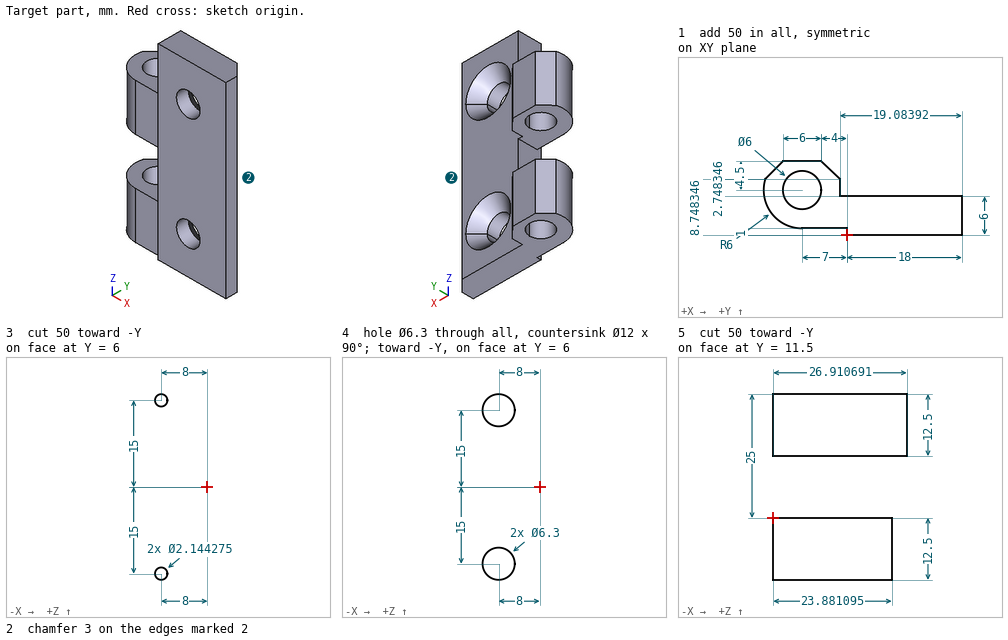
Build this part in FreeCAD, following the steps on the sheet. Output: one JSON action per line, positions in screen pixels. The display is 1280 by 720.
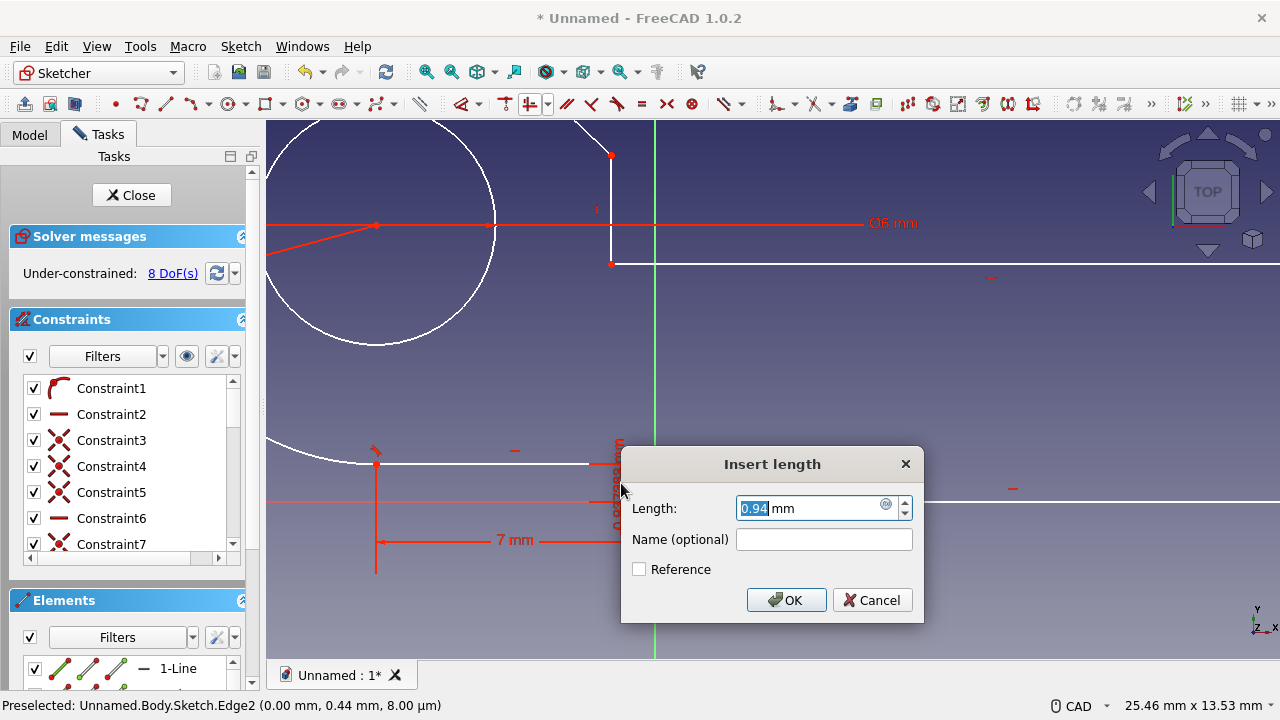
{"action": "type", "text": "1"}
{"action": "key", "text": "Return"}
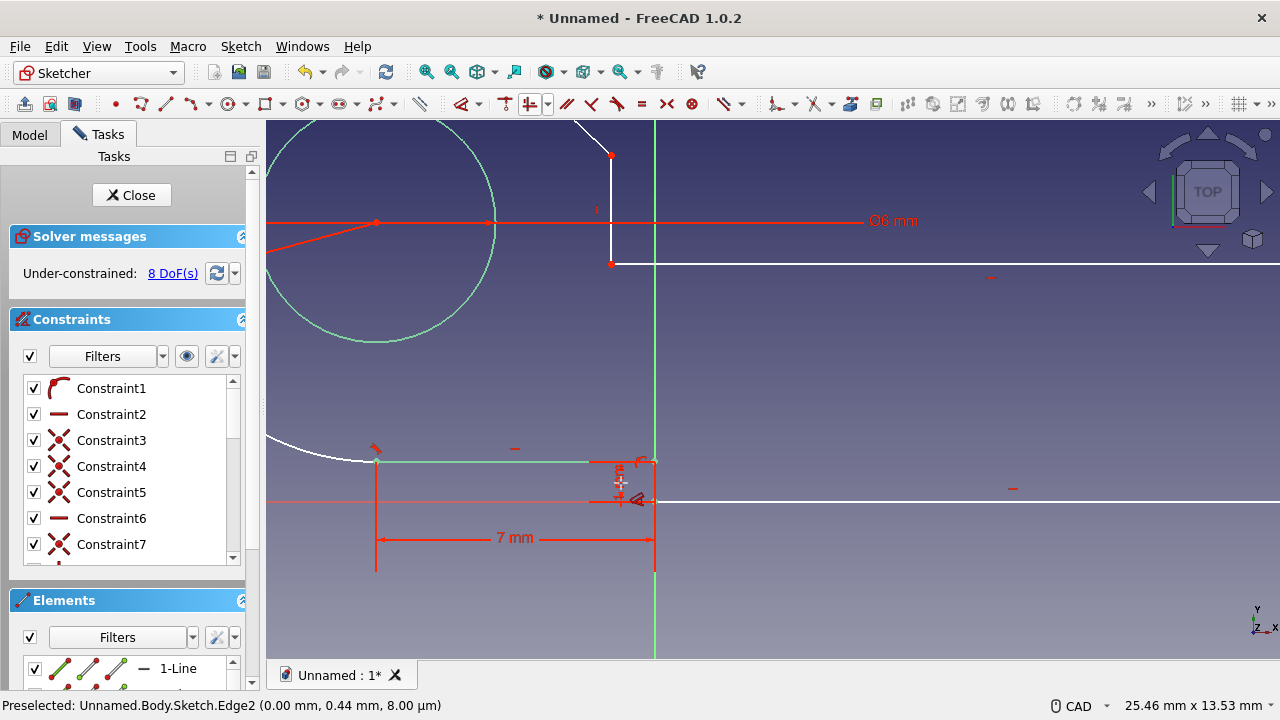
{"action": "scroll", "coordinate": [659, 485], "scroll_direction": "down", "scroll_amount": 4}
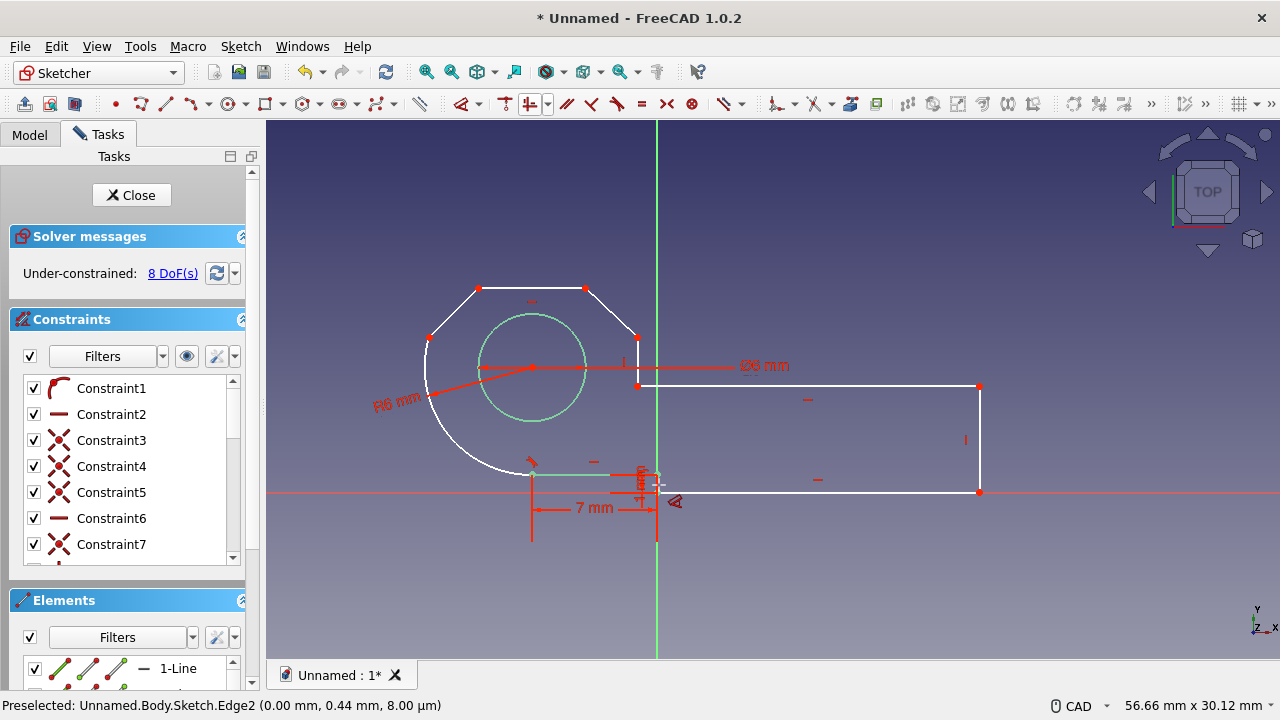
{"action": "left_click", "coordinate": [980, 461]}
{"action": "left_click", "coordinate": [1014, 439]}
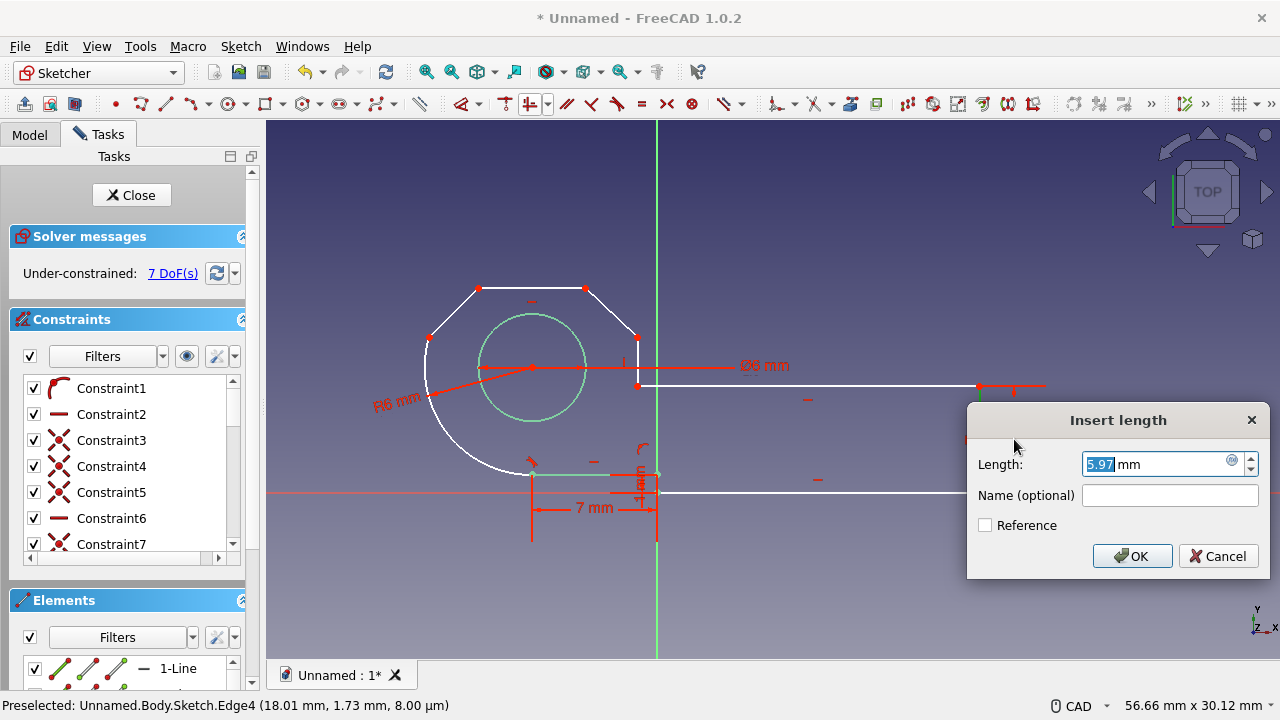
{"action": "type", "text": "6"}
{"action": "key", "text": "Return"}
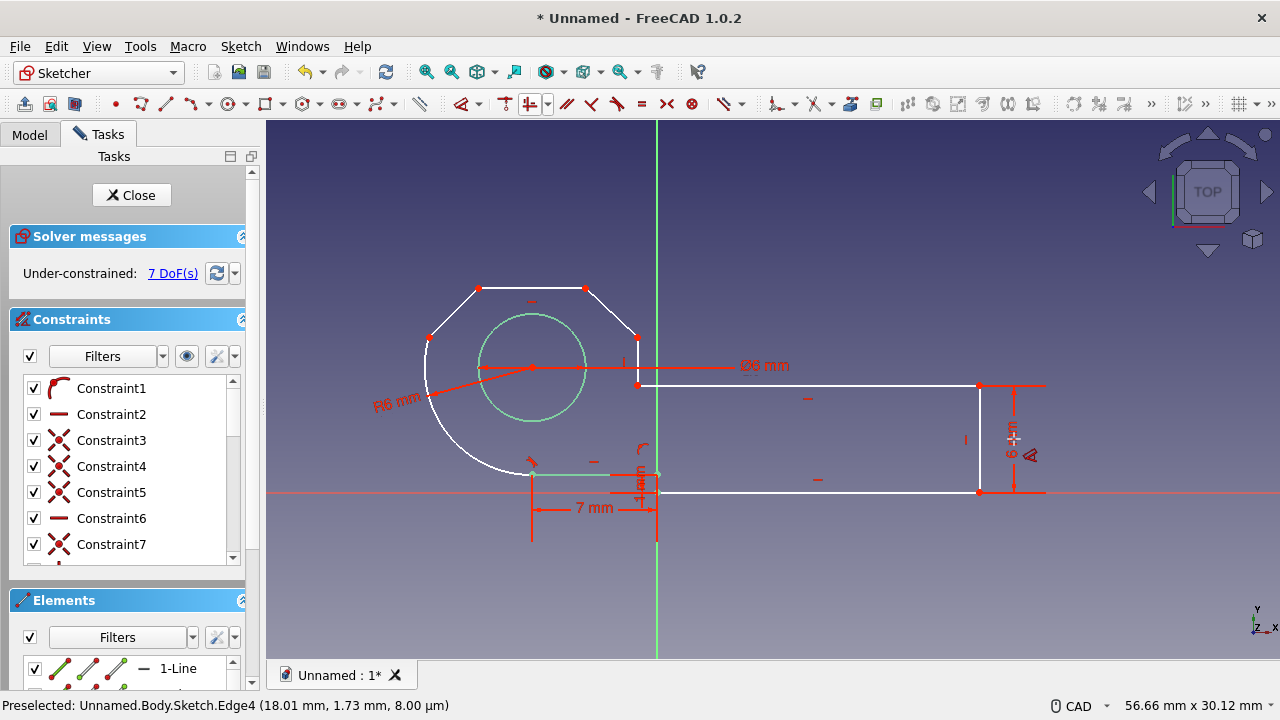
{"action": "left_click", "coordinate": [554, 288]}
{"action": "left_click", "coordinate": [532, 254]}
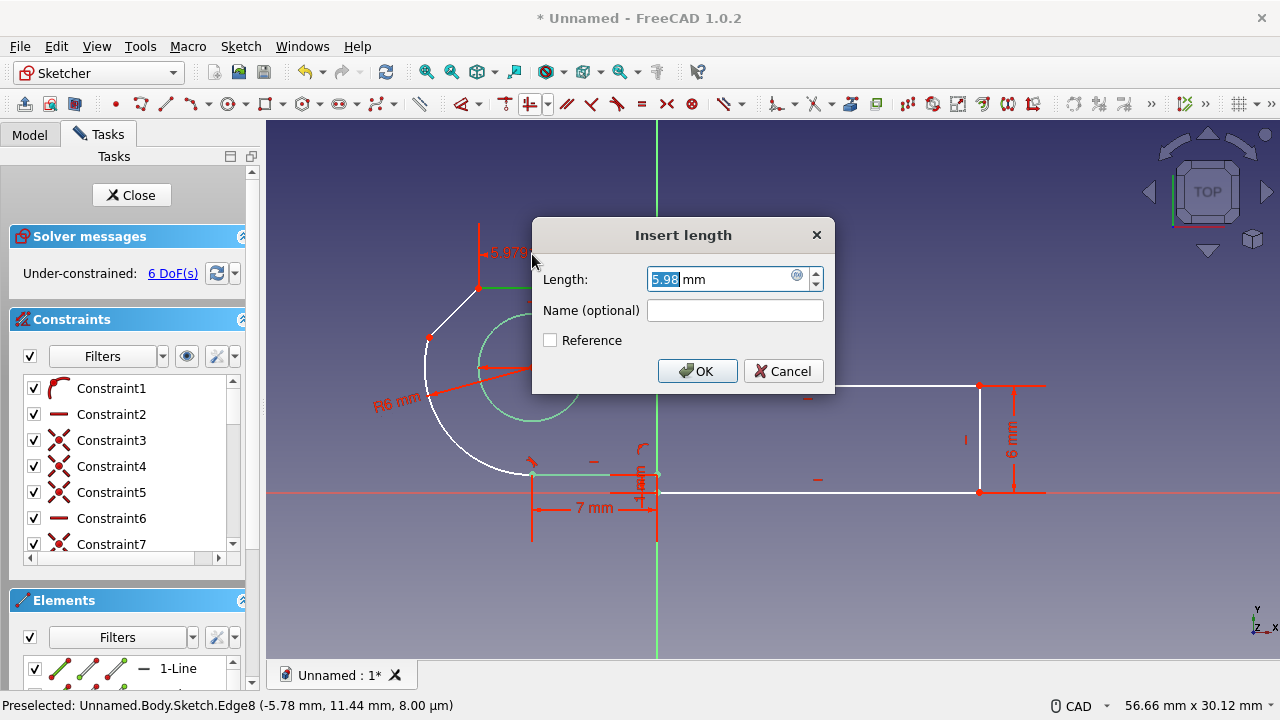
{"action": "type", "text": "6"}
{"action": "key", "text": "Return"}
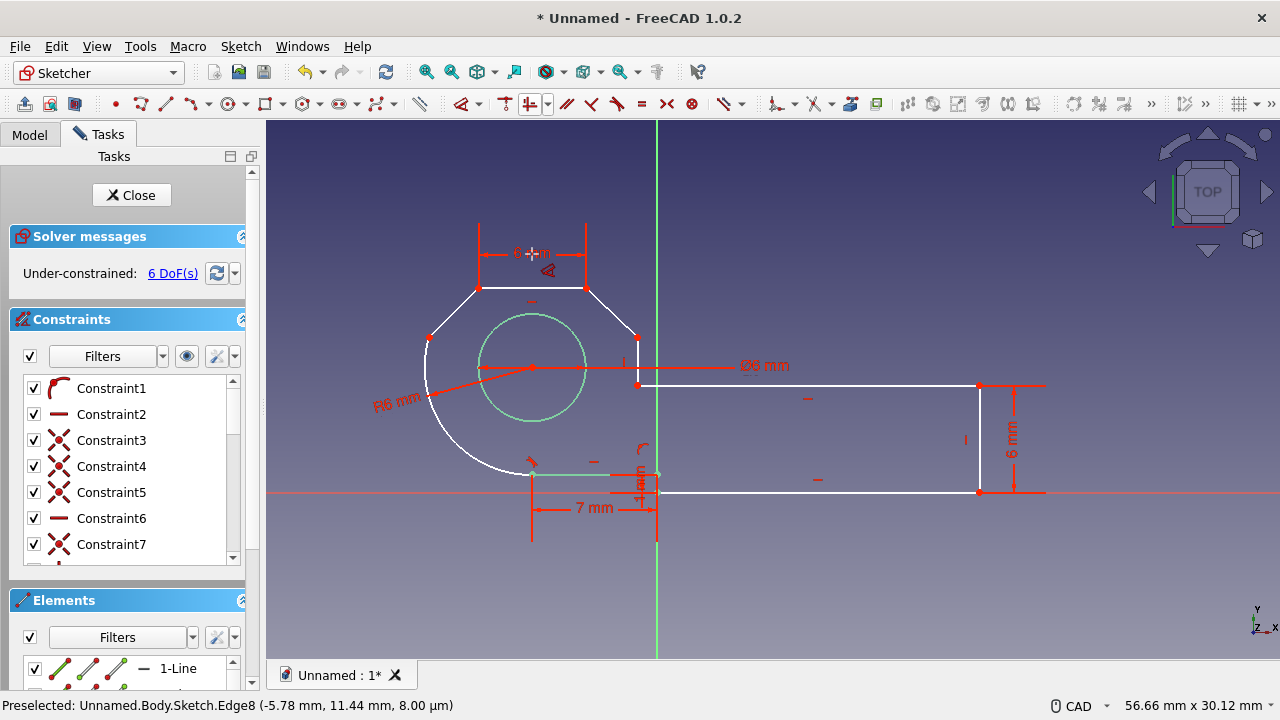
{"action": "left_click", "coordinate": [754, 493]}
{"action": "left_click", "coordinate": [819, 527]}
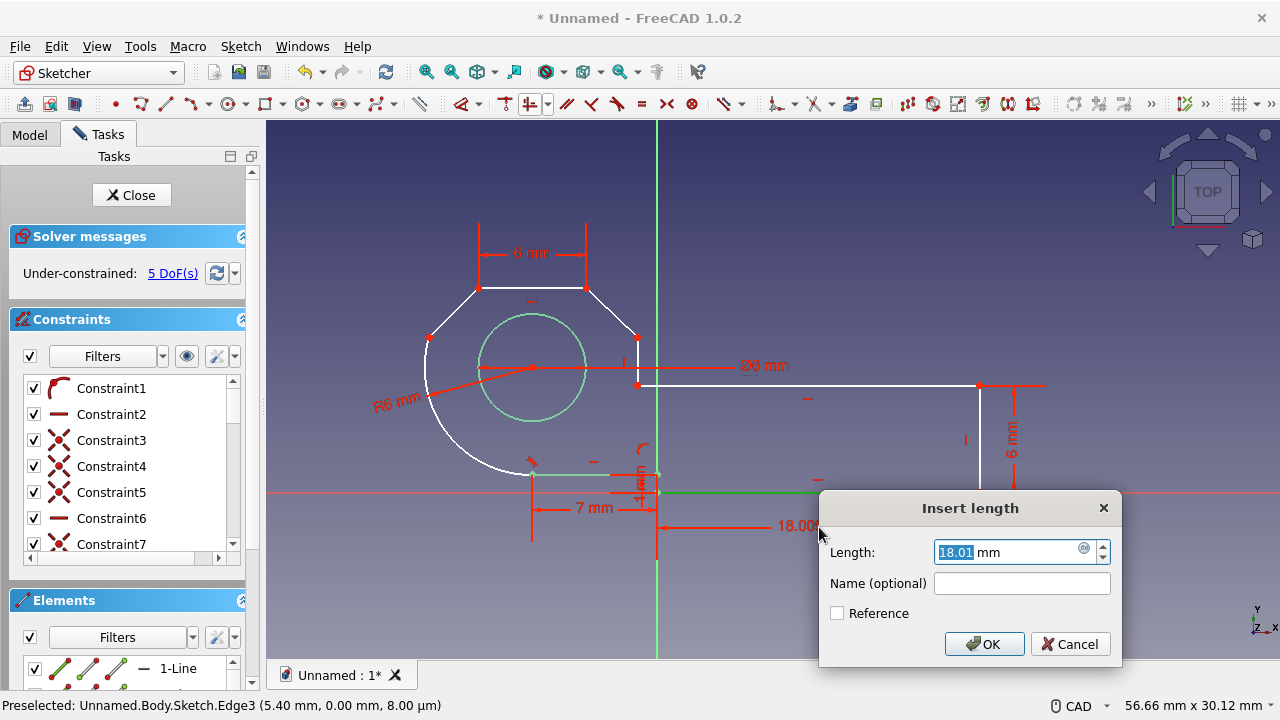
{"action": "type", "text": "18"}
{"action": "key", "text": "Return"}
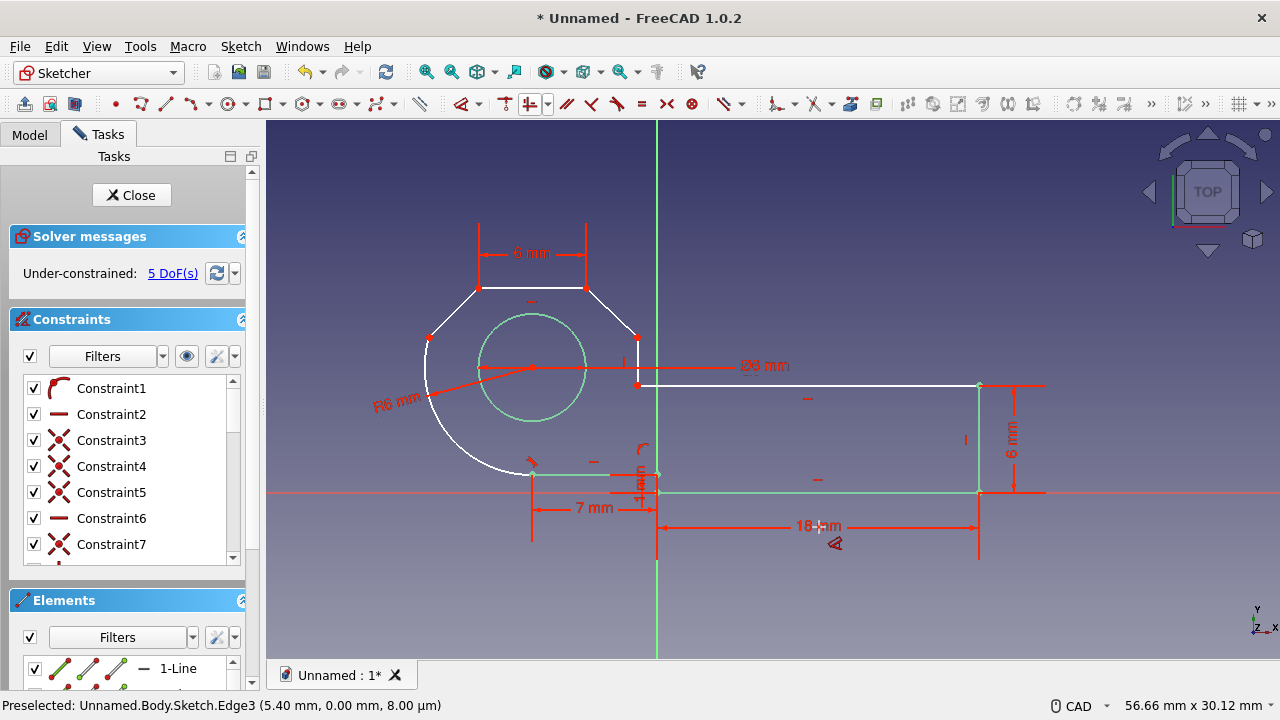
{"action": "left_click", "coordinate": [586, 288]}
{"action": "left_click", "coordinate": [622, 254]}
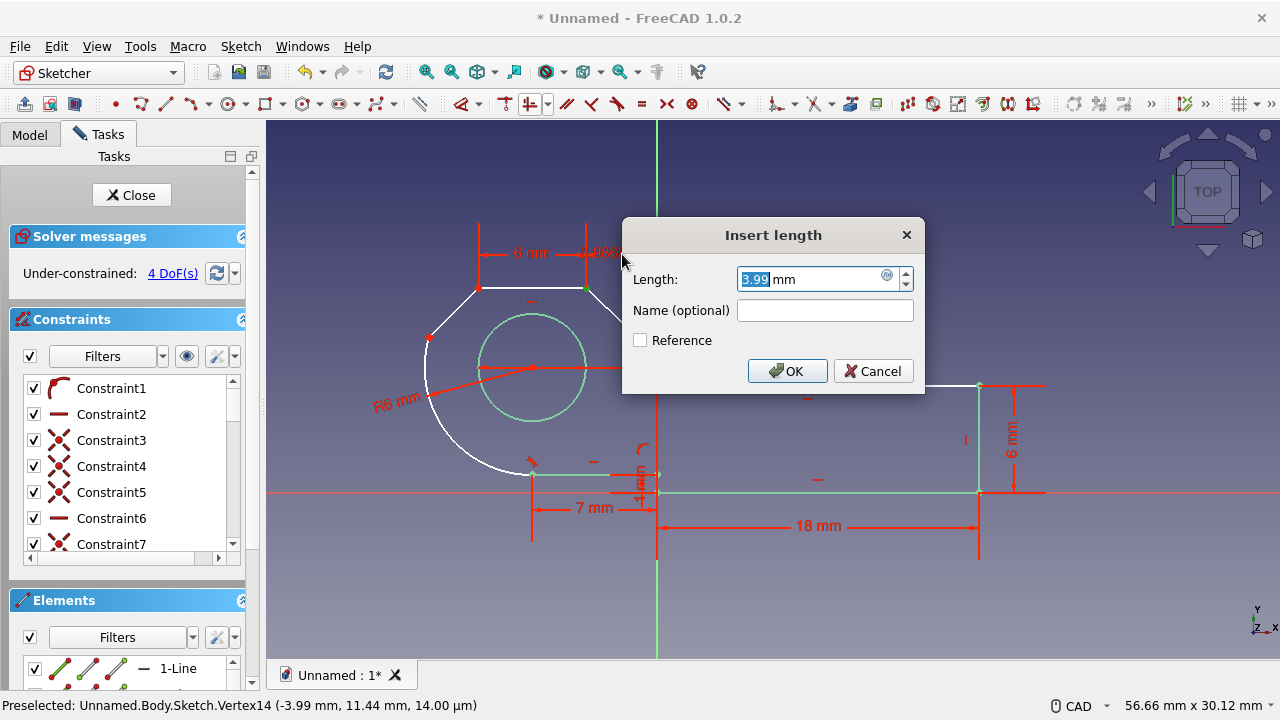
{"action": "type", "text": "4"}
{"action": "key", "text": "Return"}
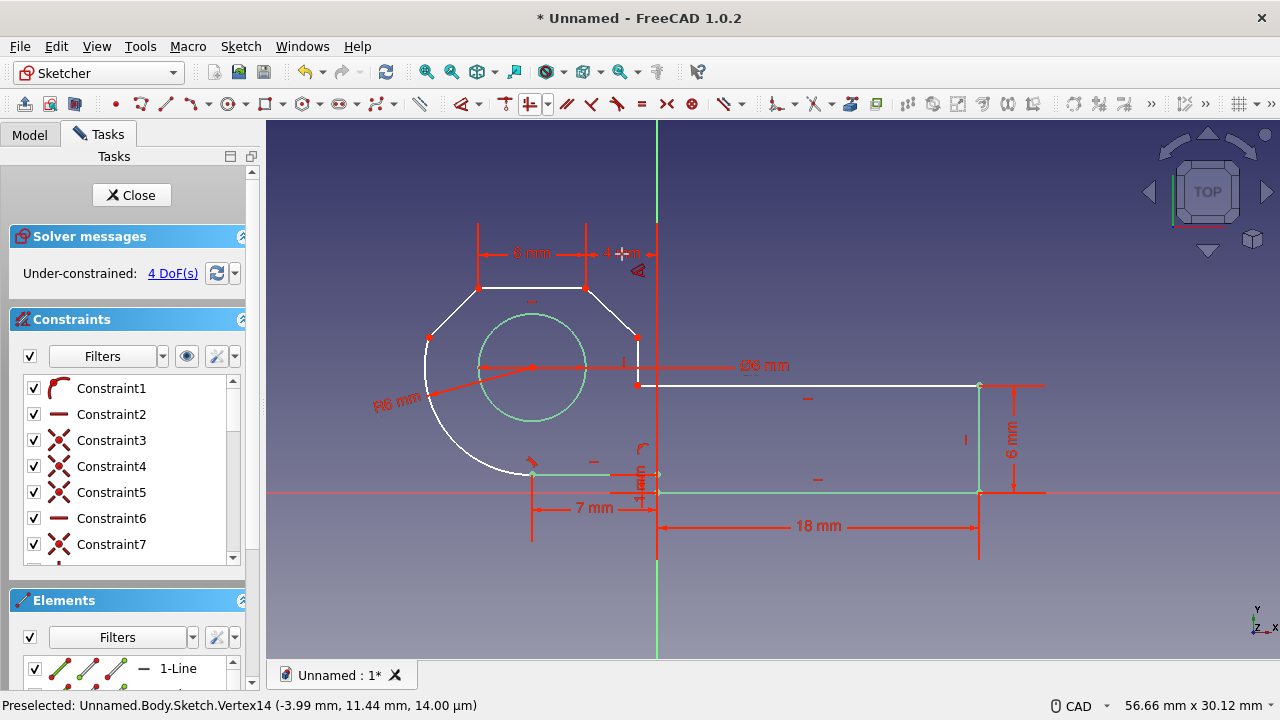
{"action": "left_click", "coordinate": [586, 288]}